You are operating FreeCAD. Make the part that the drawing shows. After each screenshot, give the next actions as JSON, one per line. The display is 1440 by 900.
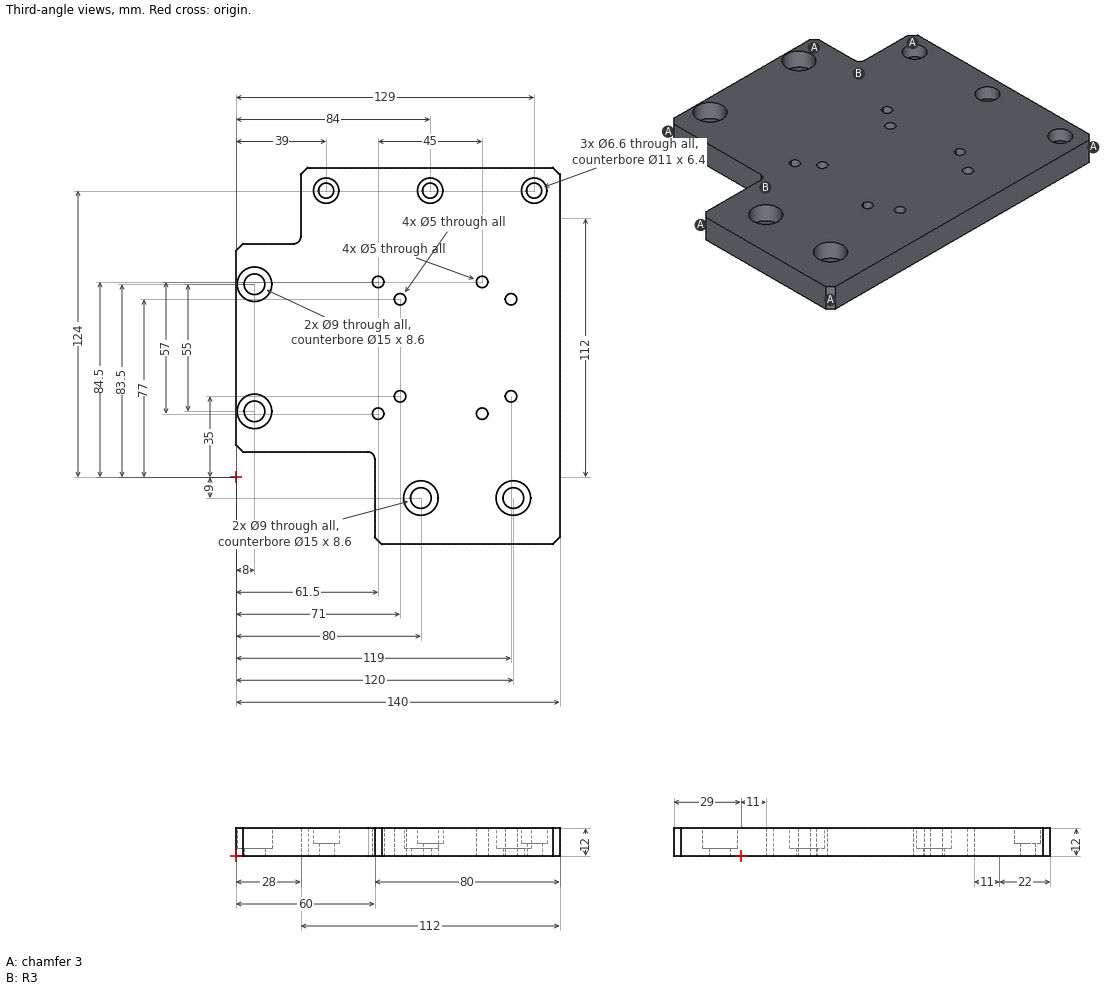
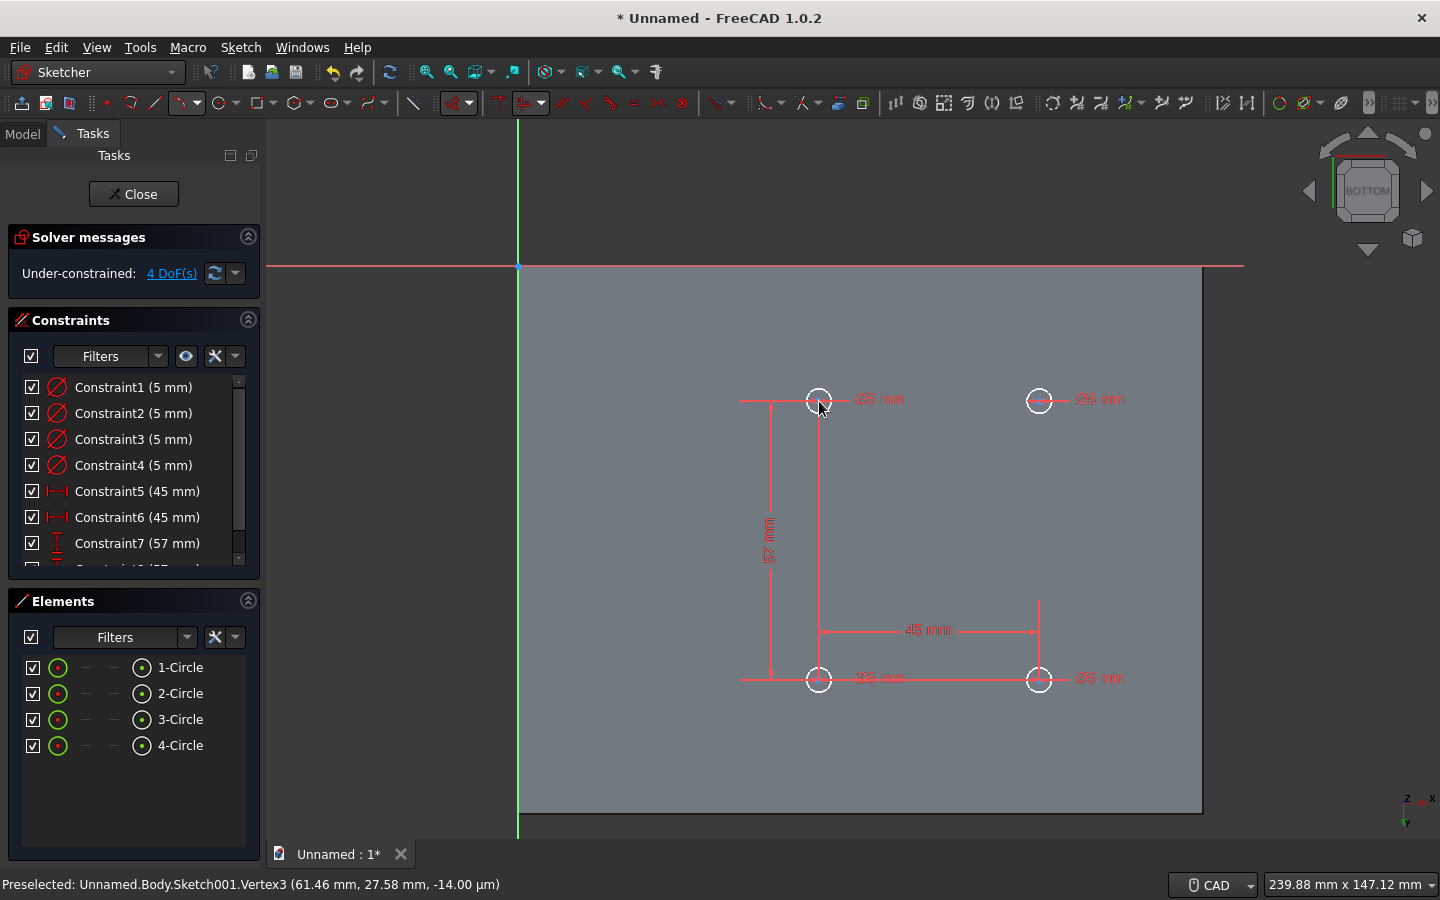
{"action": "left_click", "coordinate": [819, 401]}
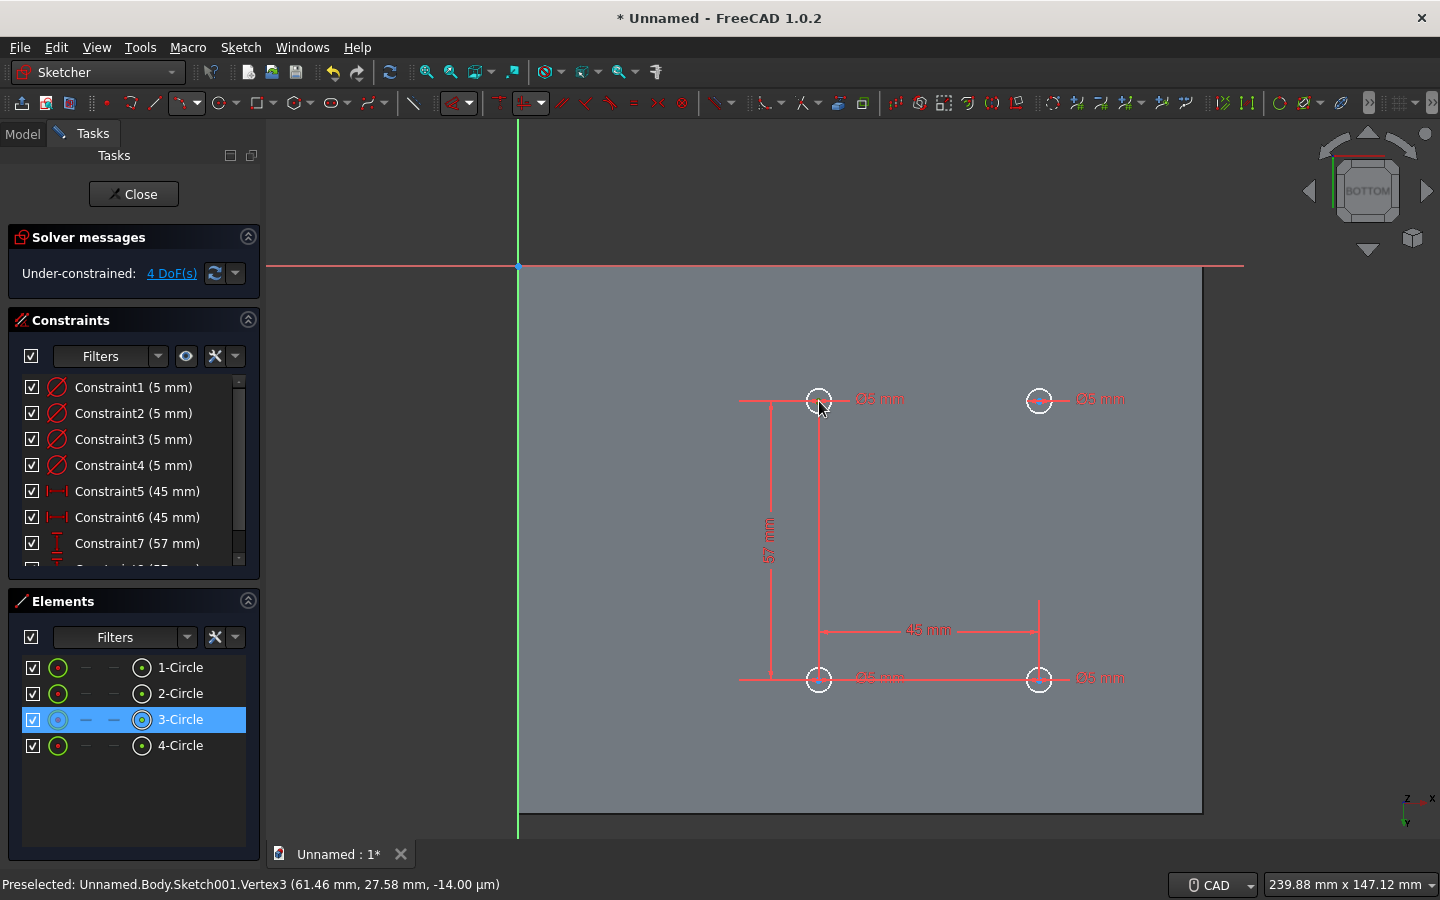
{"action": "left_click", "coordinate": [1039, 401]}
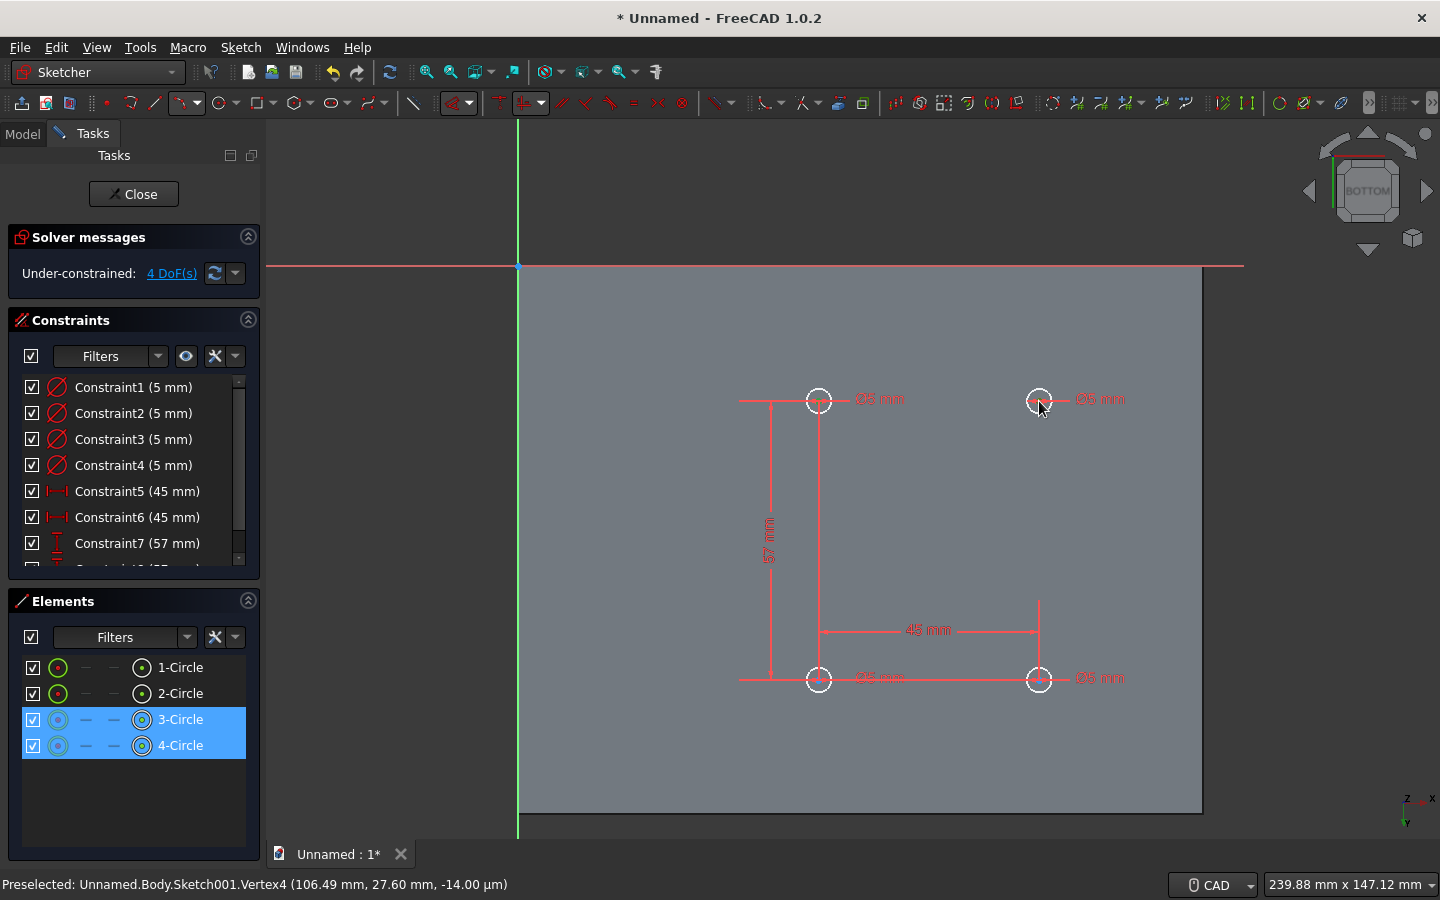
{"action": "left_click", "coordinate": [472, 104]}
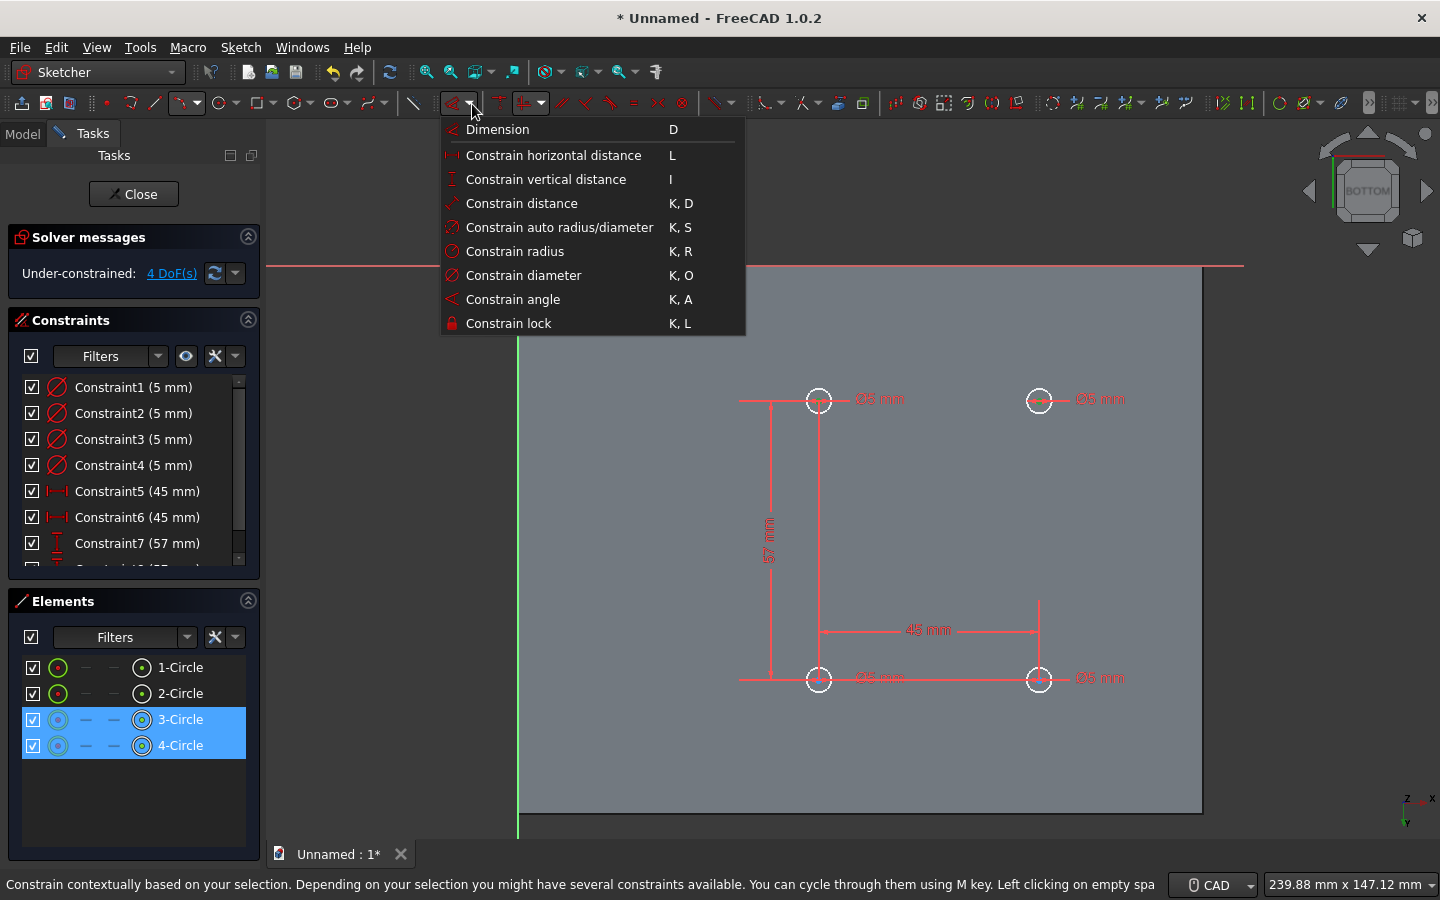
{"action": "left_click", "coordinate": [593, 155]}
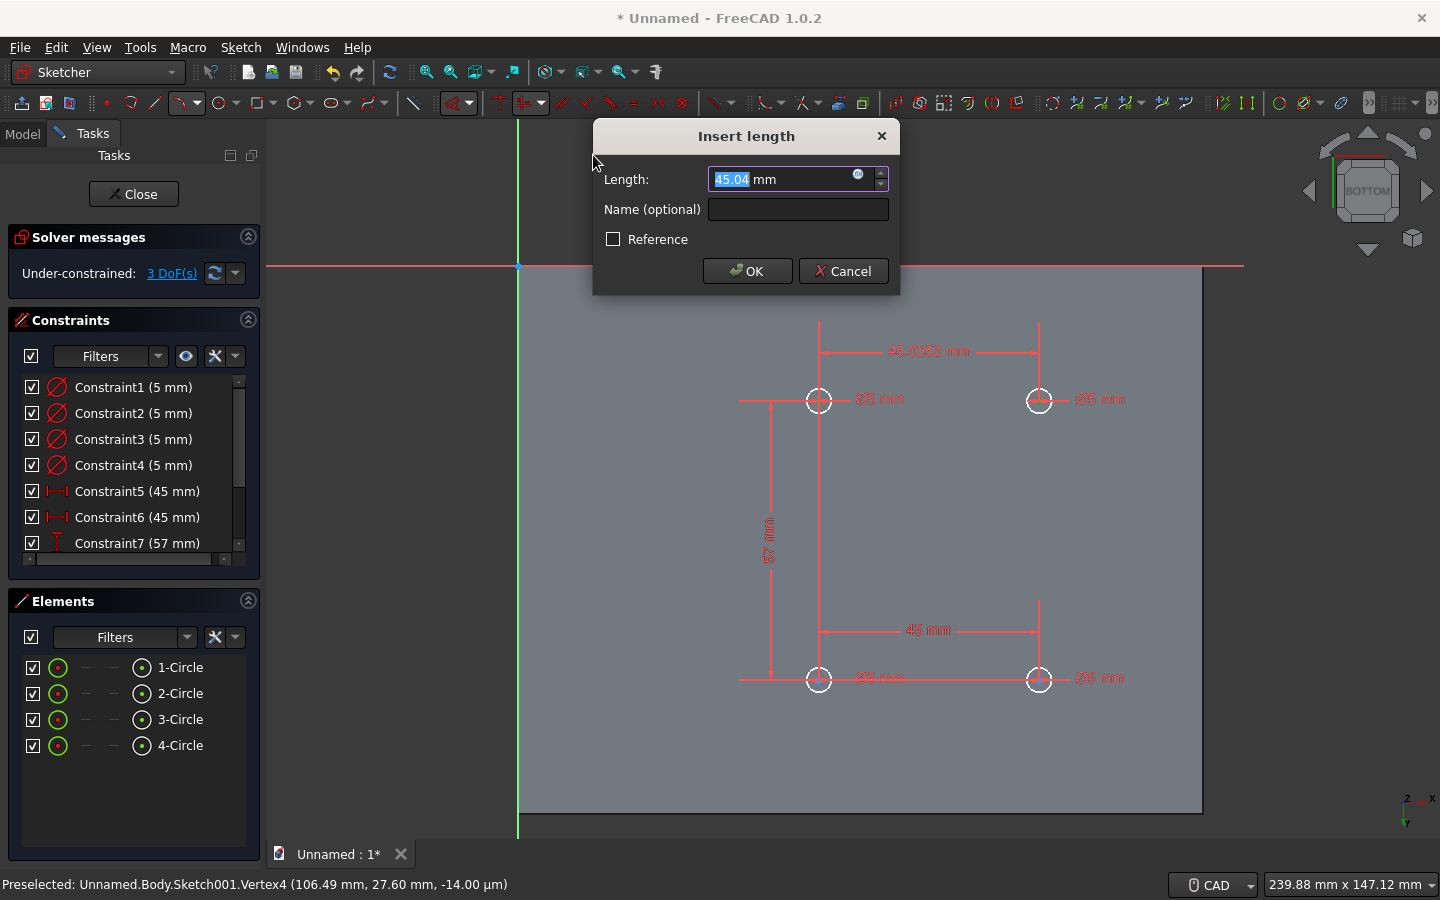
{"action": "type", "text": "45"}
{"action": "key", "text": "Return"}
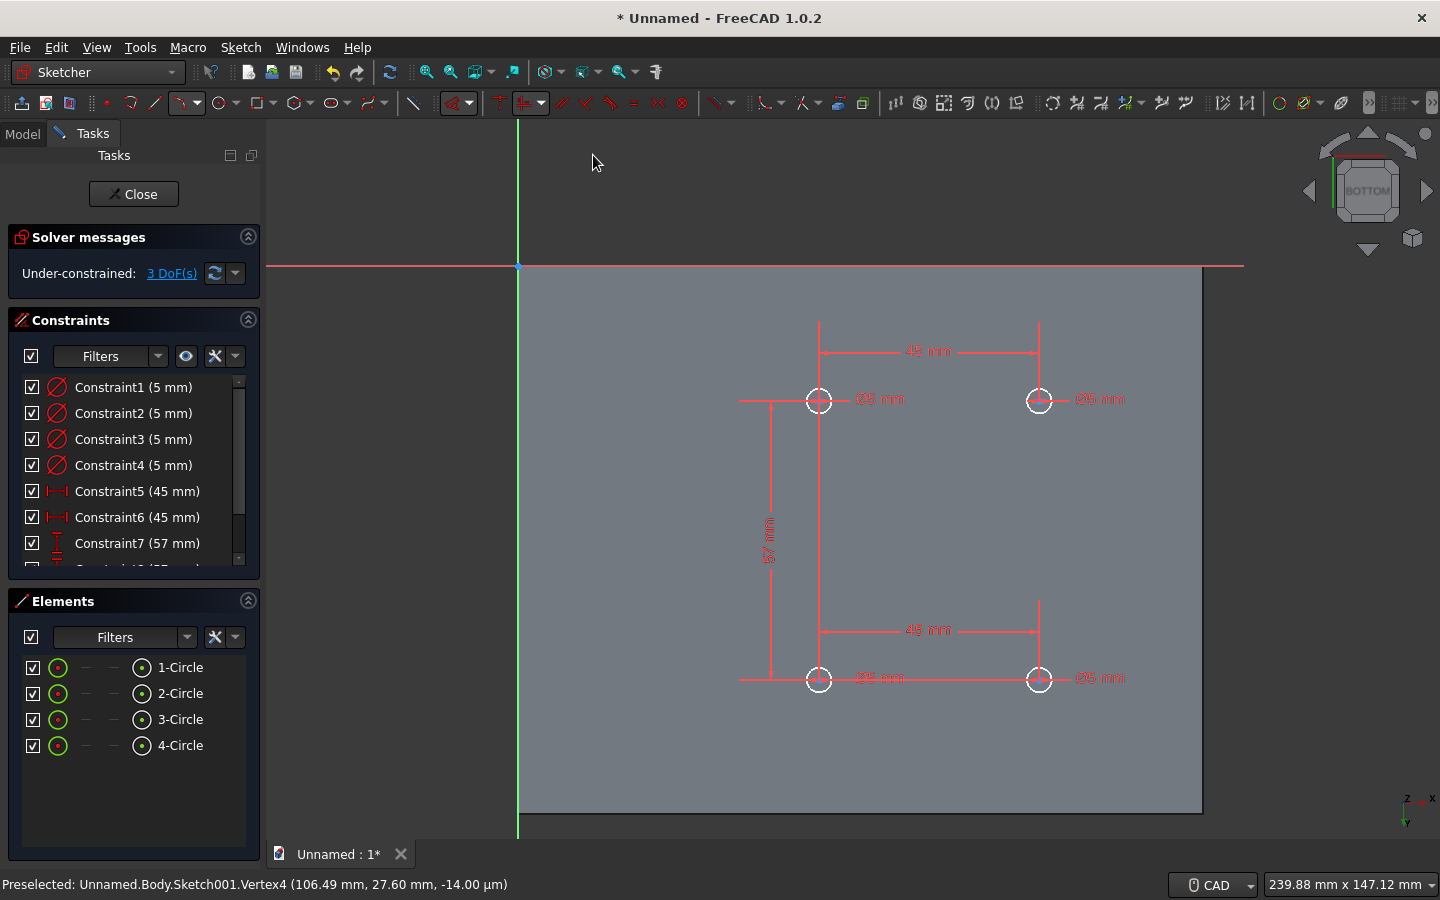
{"action": "left_click", "coordinate": [1039, 680]}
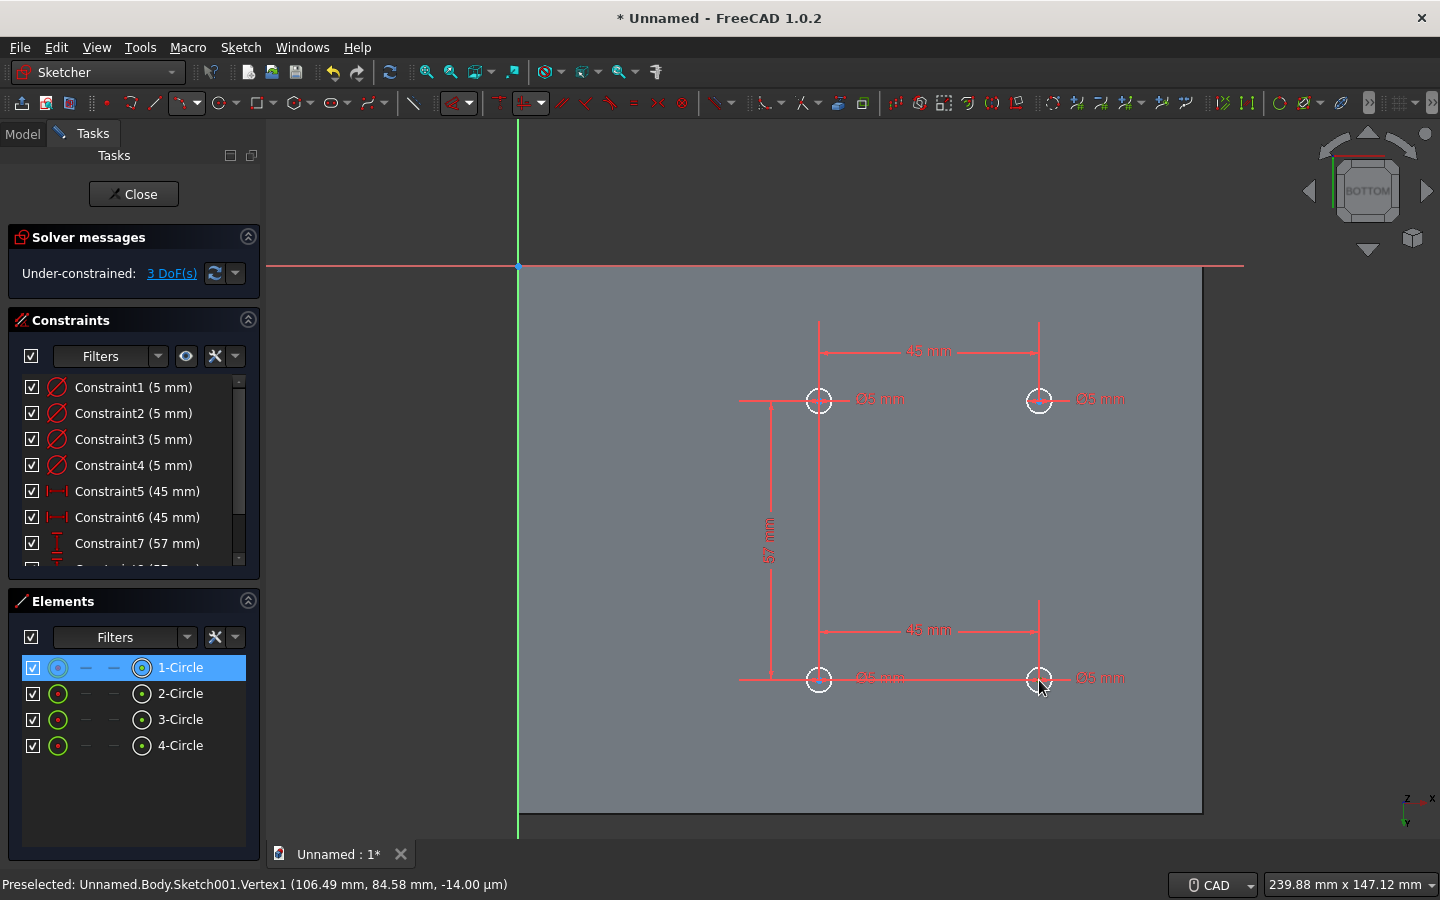
{"action": "left_click", "coordinate": [1039, 401]}